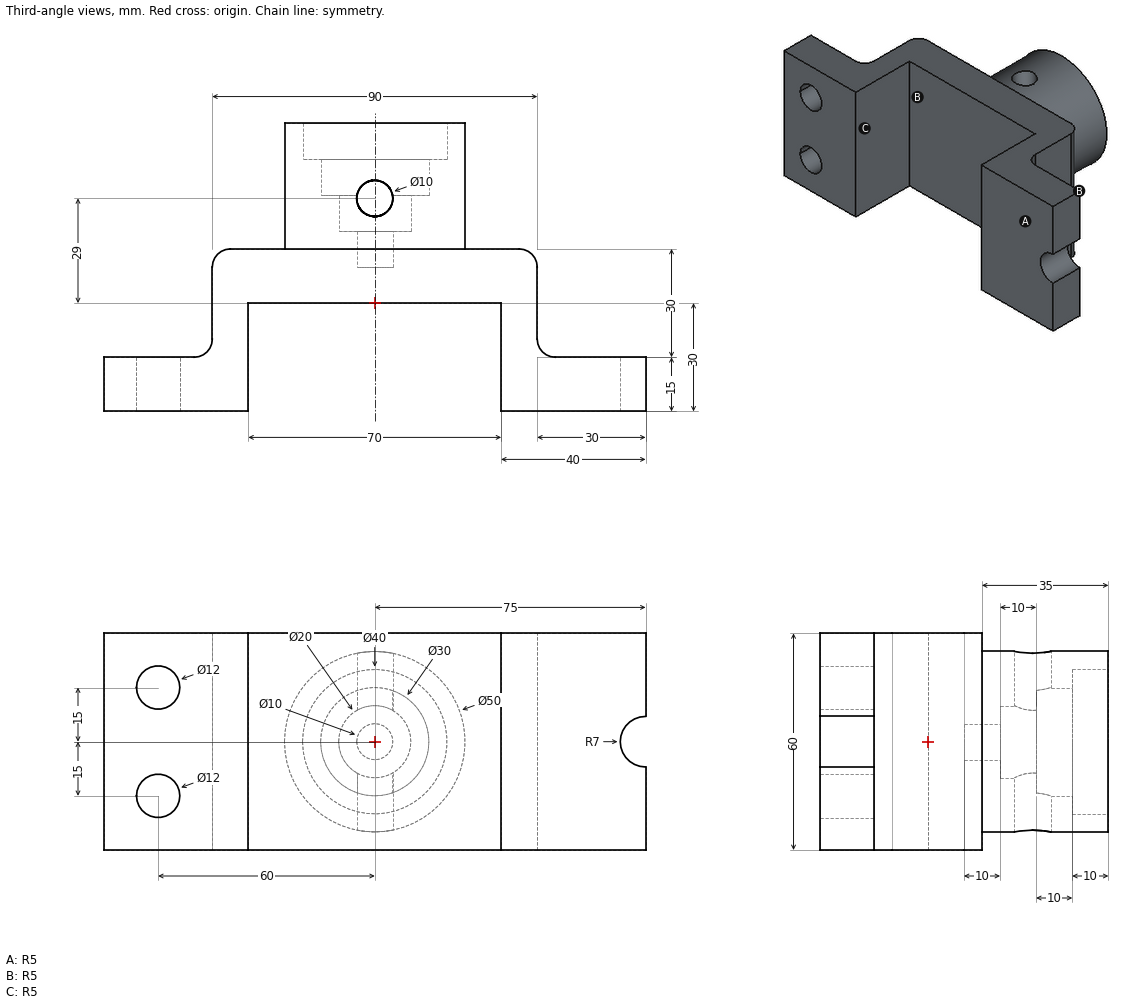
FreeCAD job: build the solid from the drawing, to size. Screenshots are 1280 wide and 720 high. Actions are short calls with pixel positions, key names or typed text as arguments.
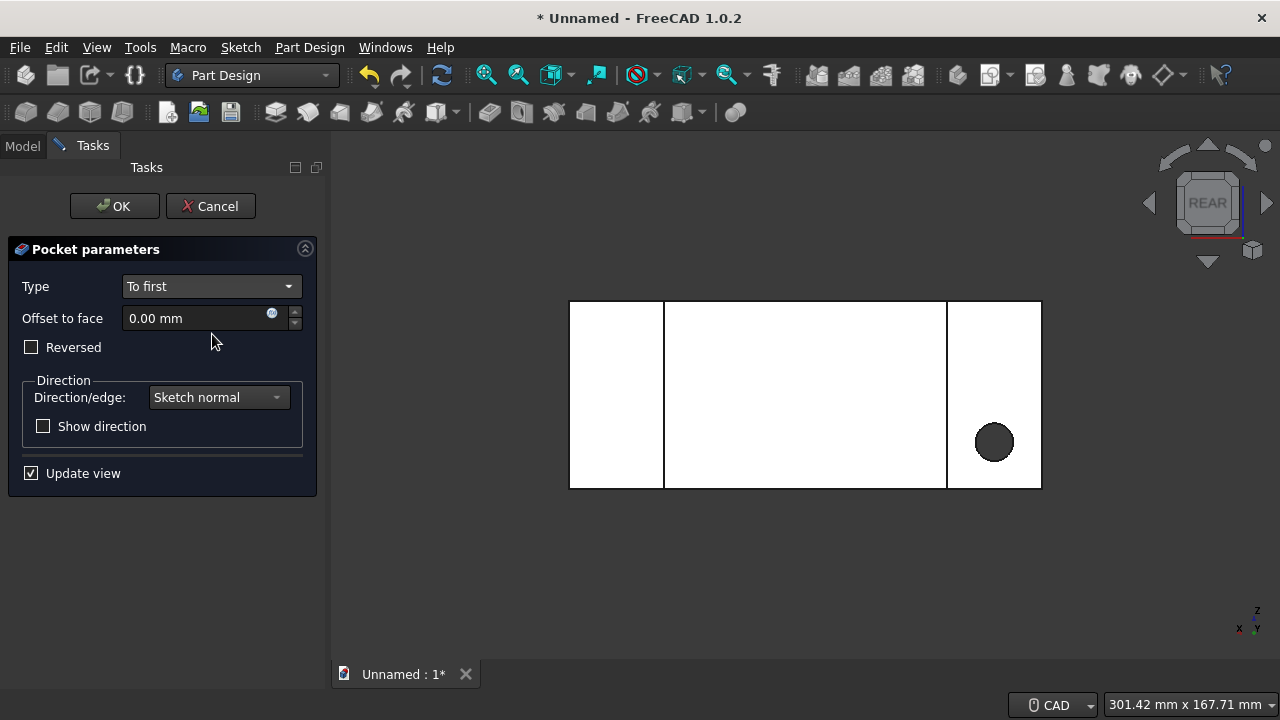
click(115, 206)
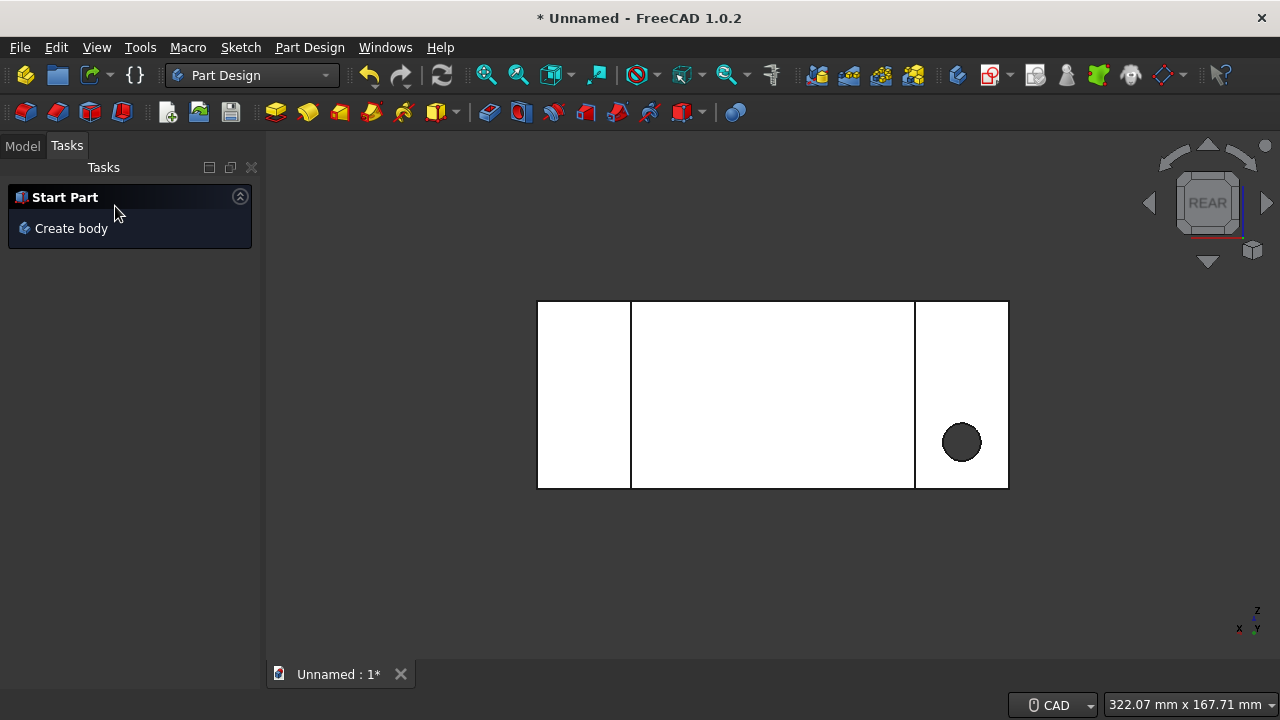
click(584, 367)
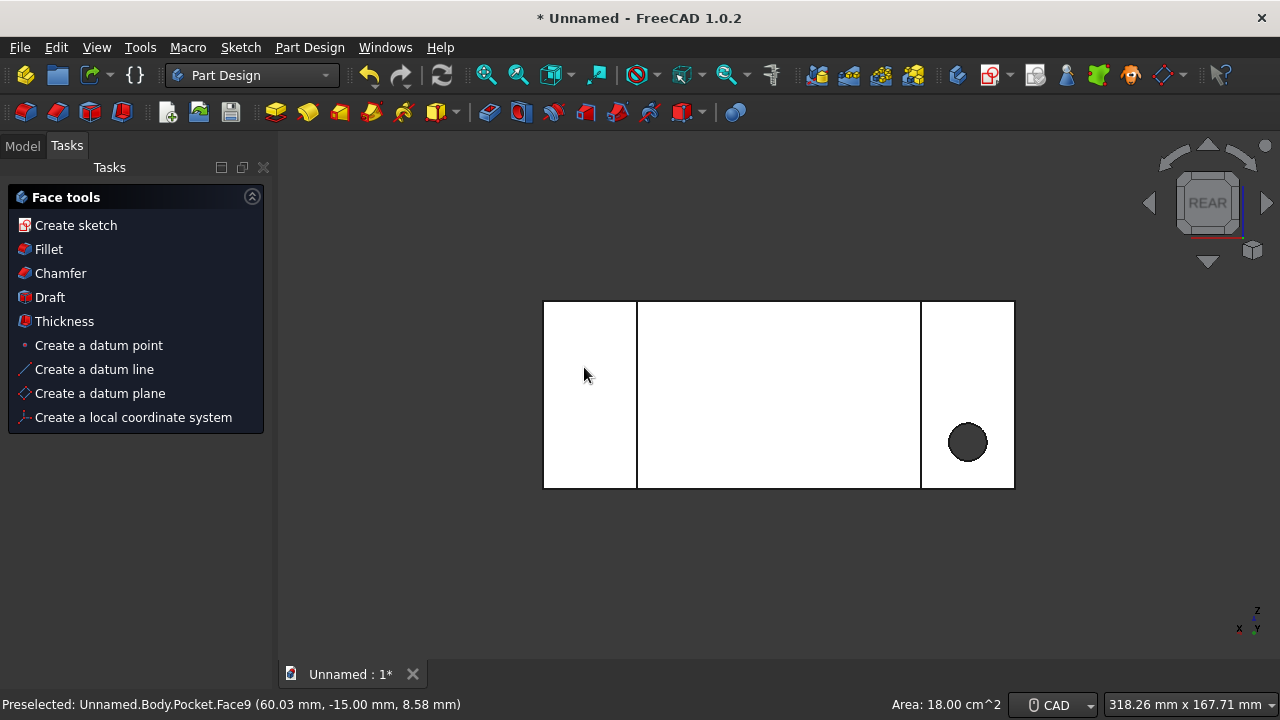
click(990, 76)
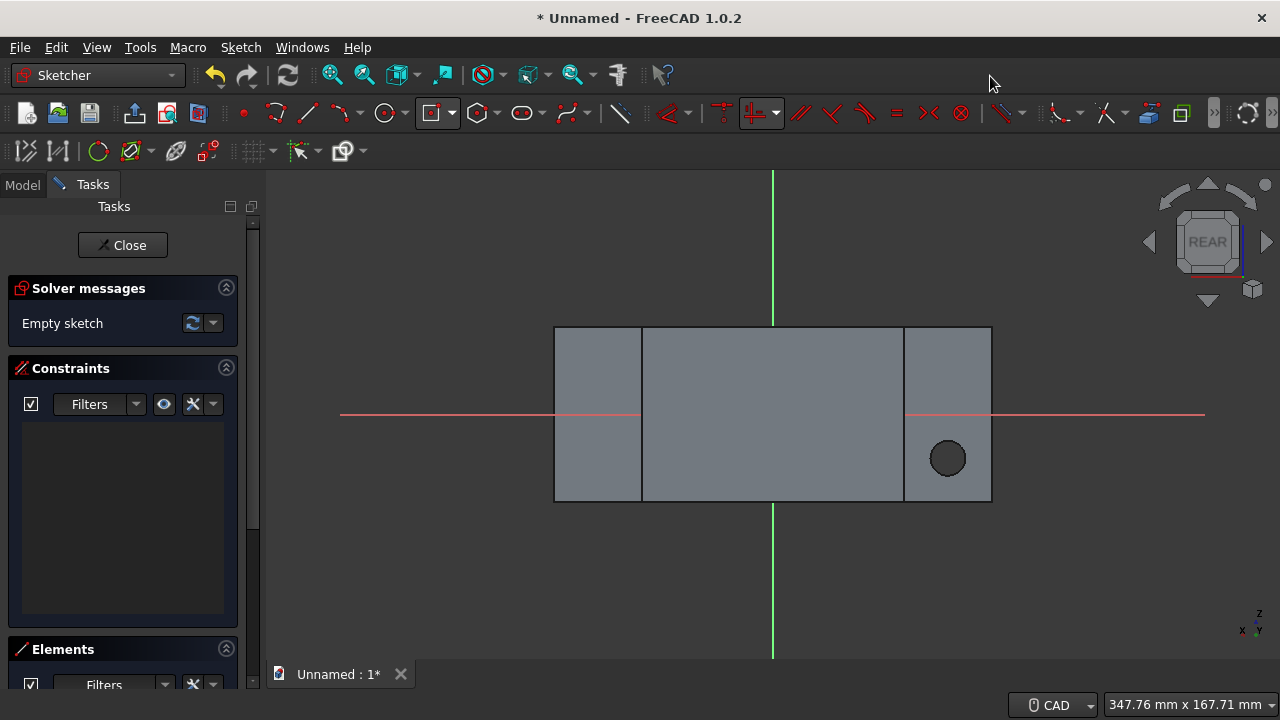
scroll(978, 365, up, 11)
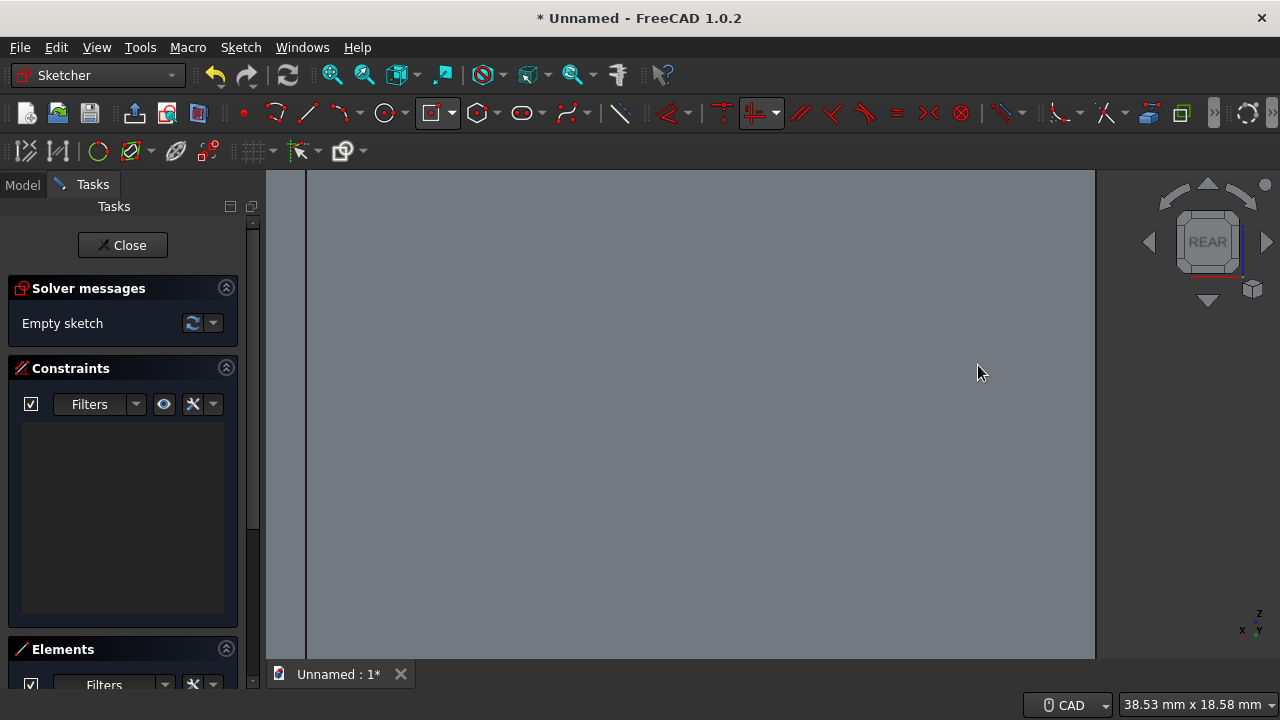
click(386, 114)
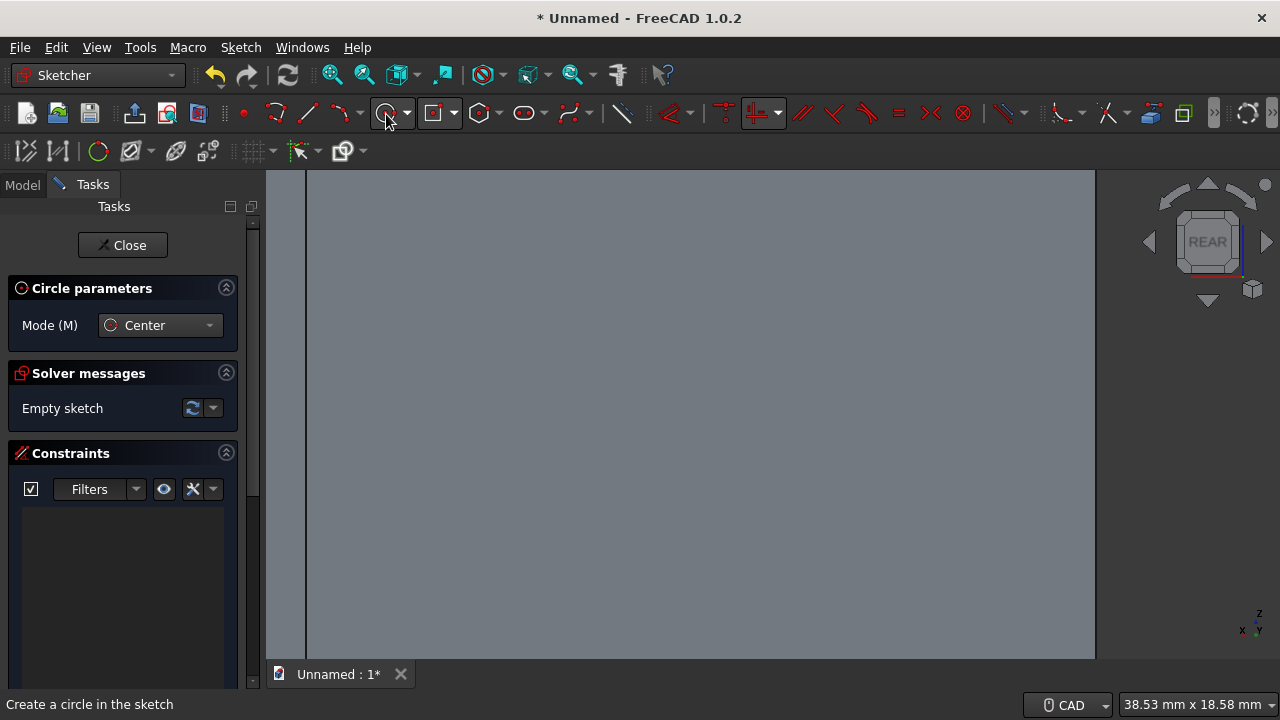
click(701, 414)
click(813, 302)
key(Escape)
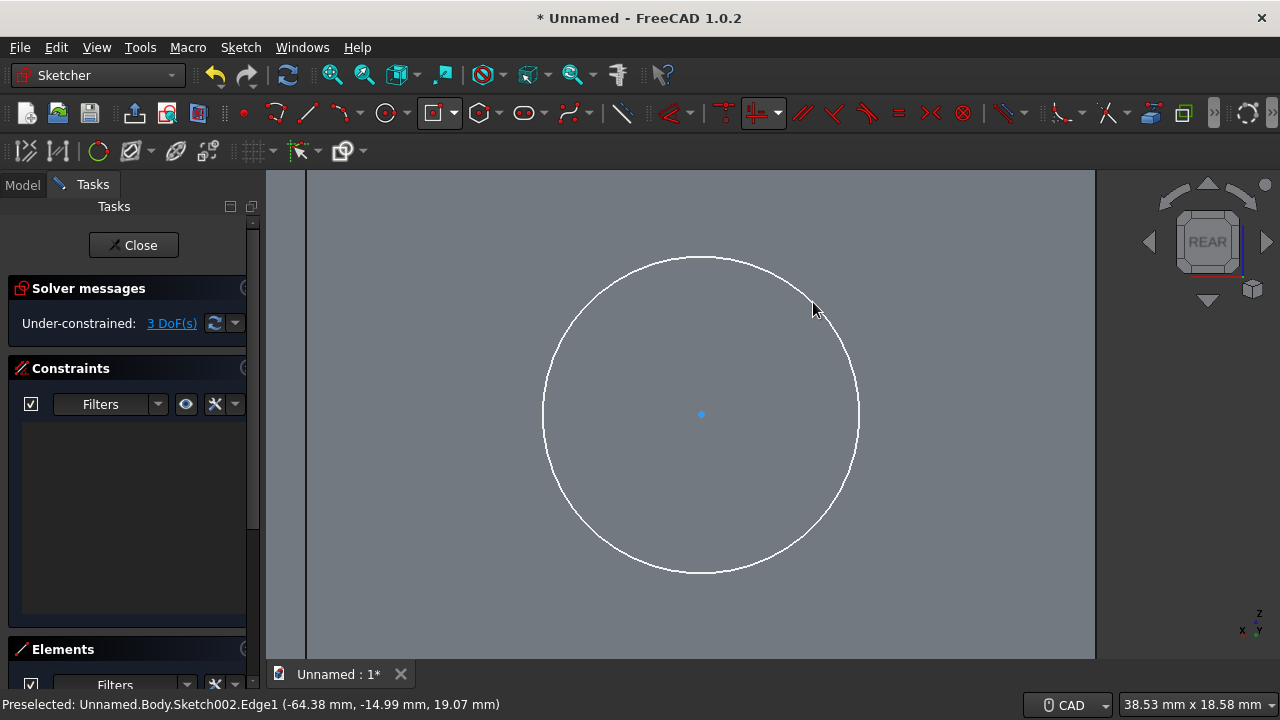
click(670, 114)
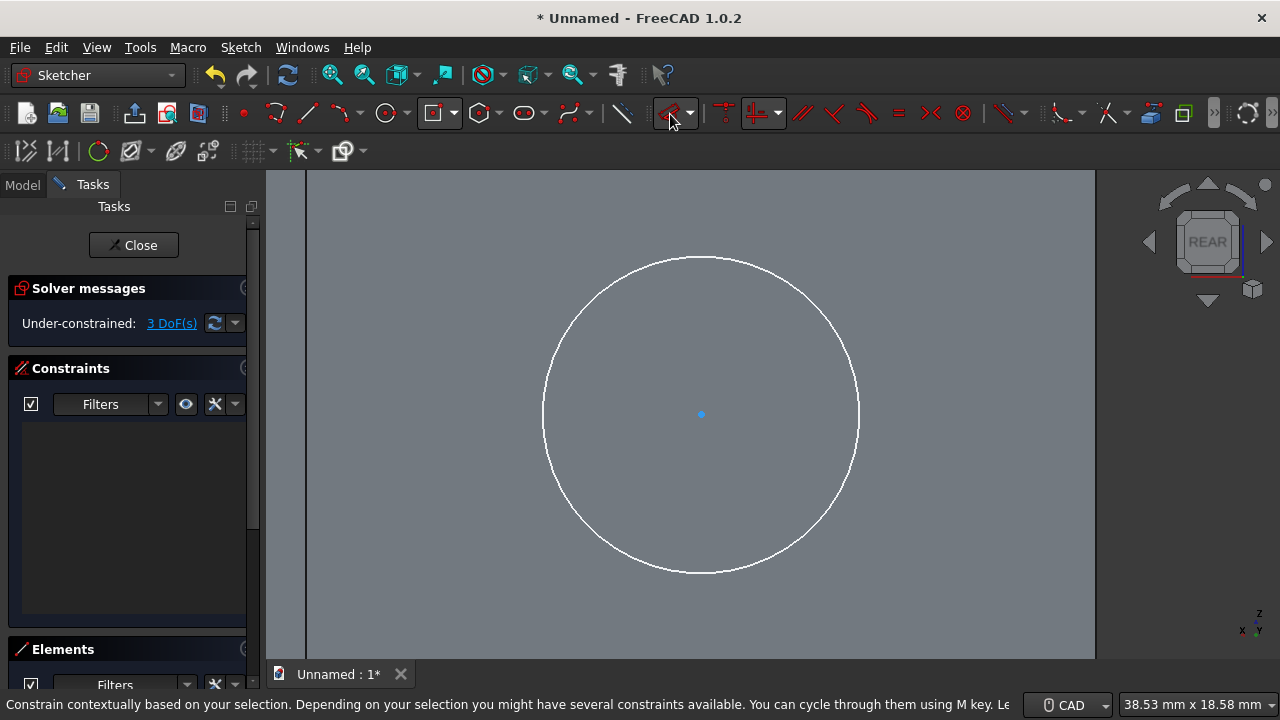
click(813, 303)
click(836, 280)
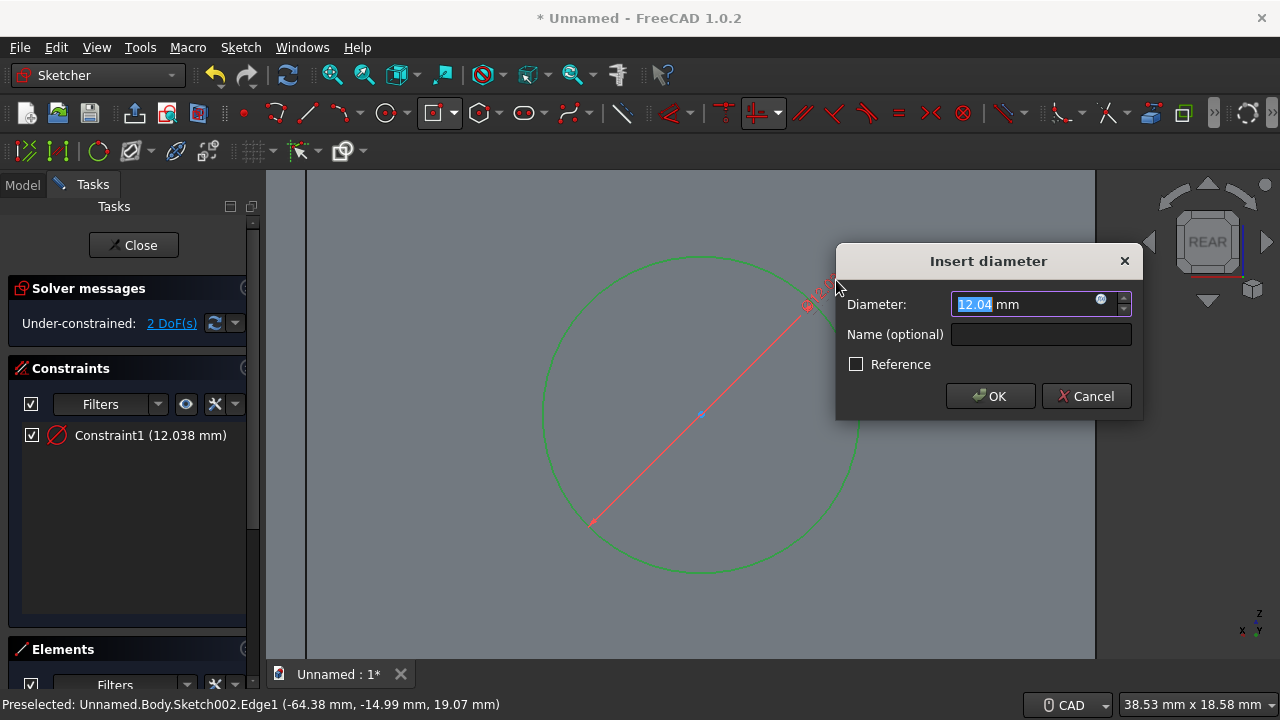
text(12)
key(Return)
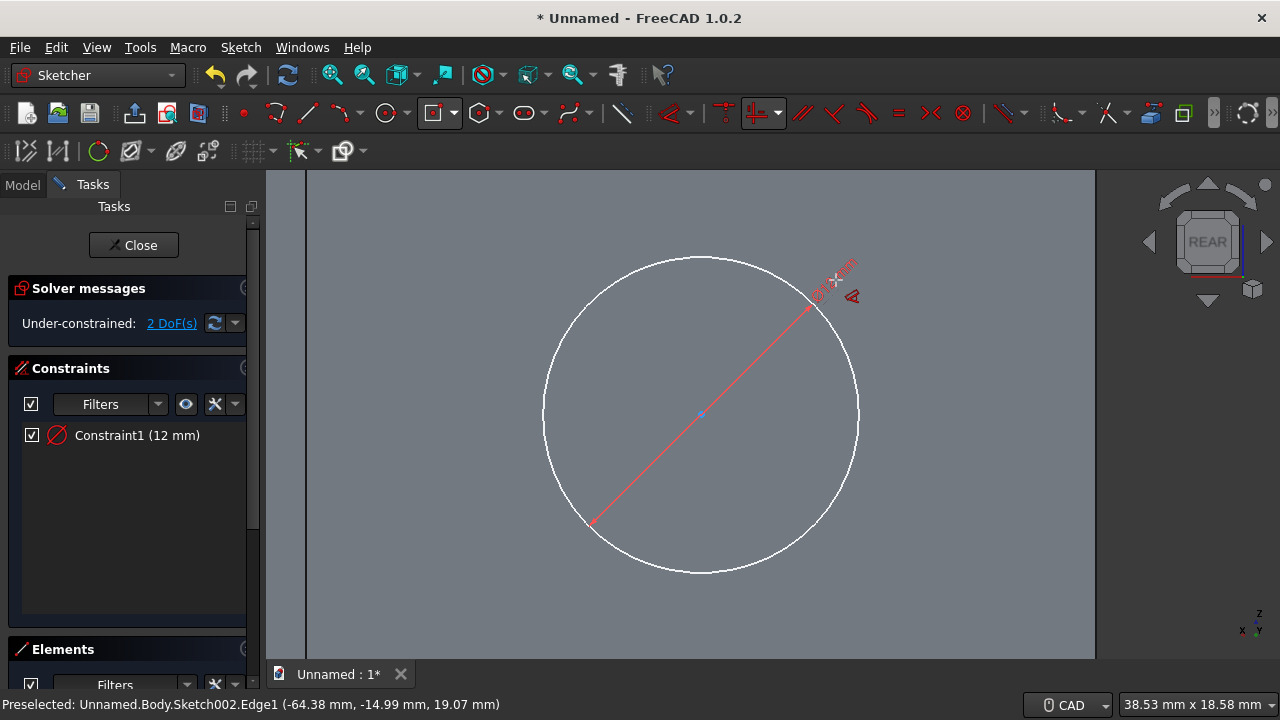
click(701, 415)
click(497, 381)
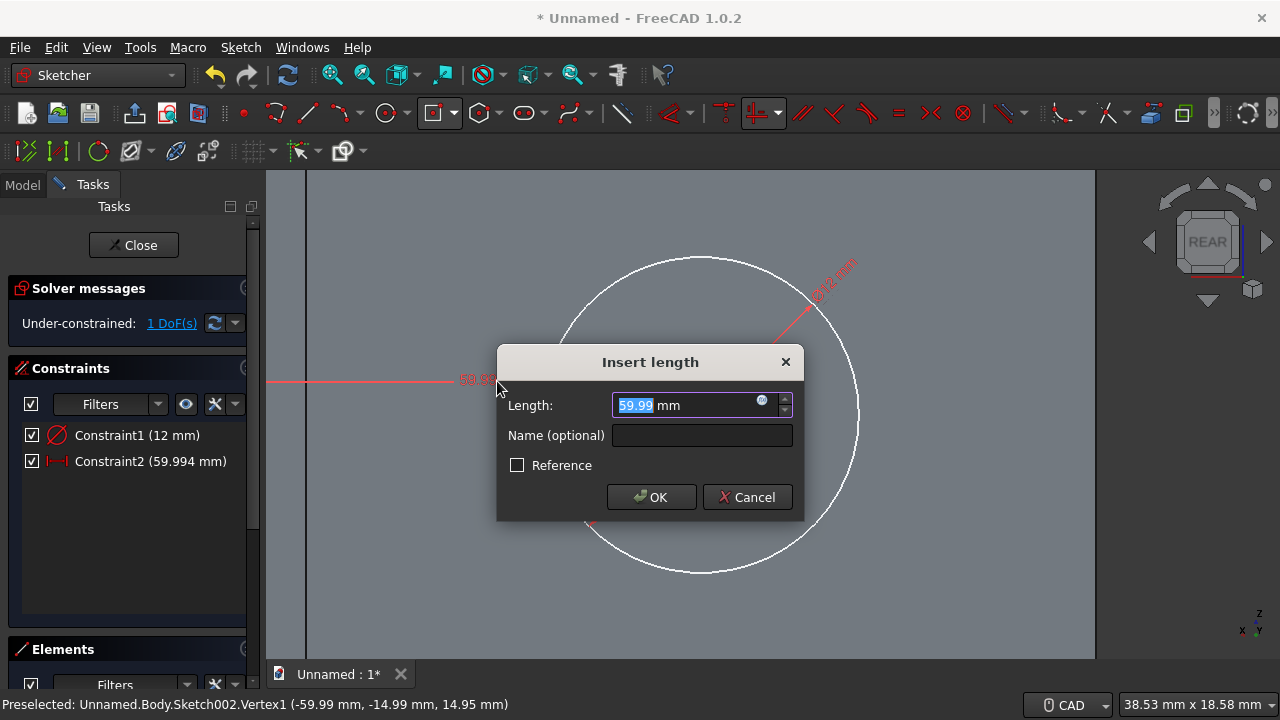
text(60)
key(Return)